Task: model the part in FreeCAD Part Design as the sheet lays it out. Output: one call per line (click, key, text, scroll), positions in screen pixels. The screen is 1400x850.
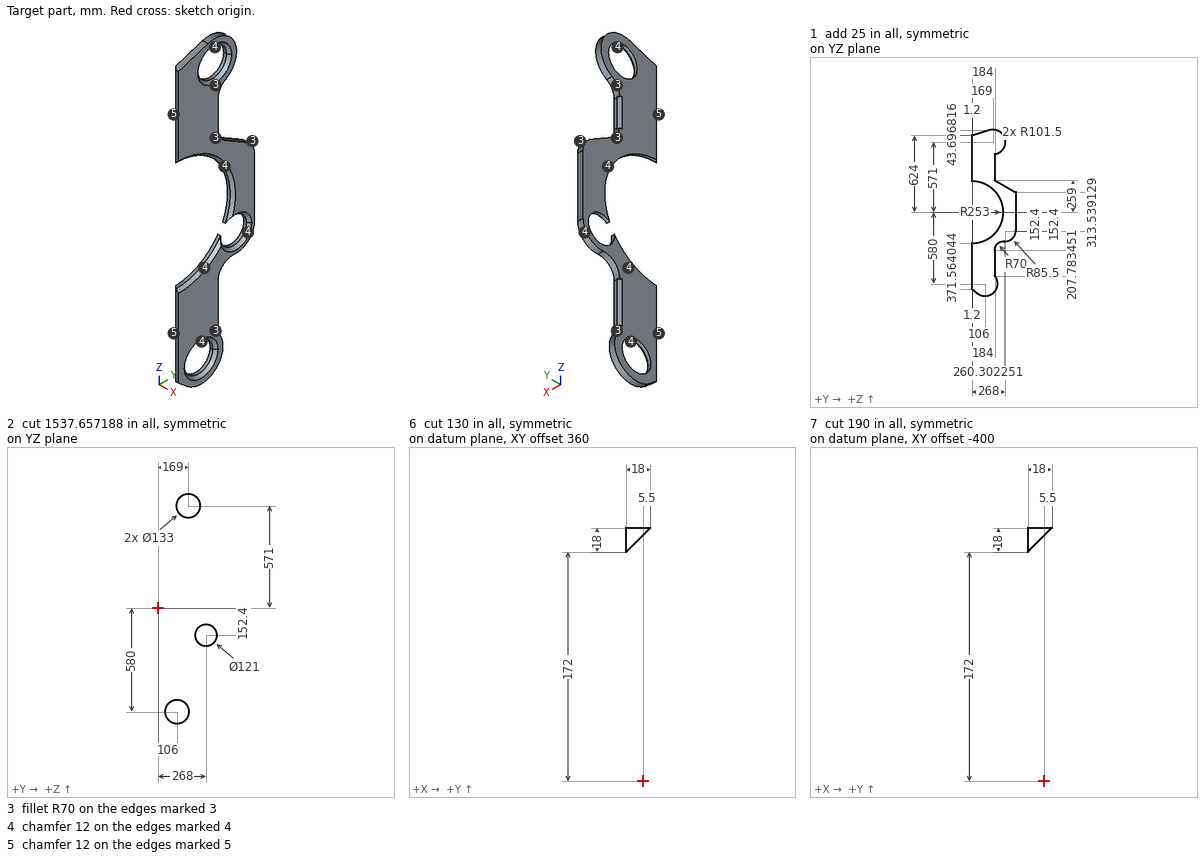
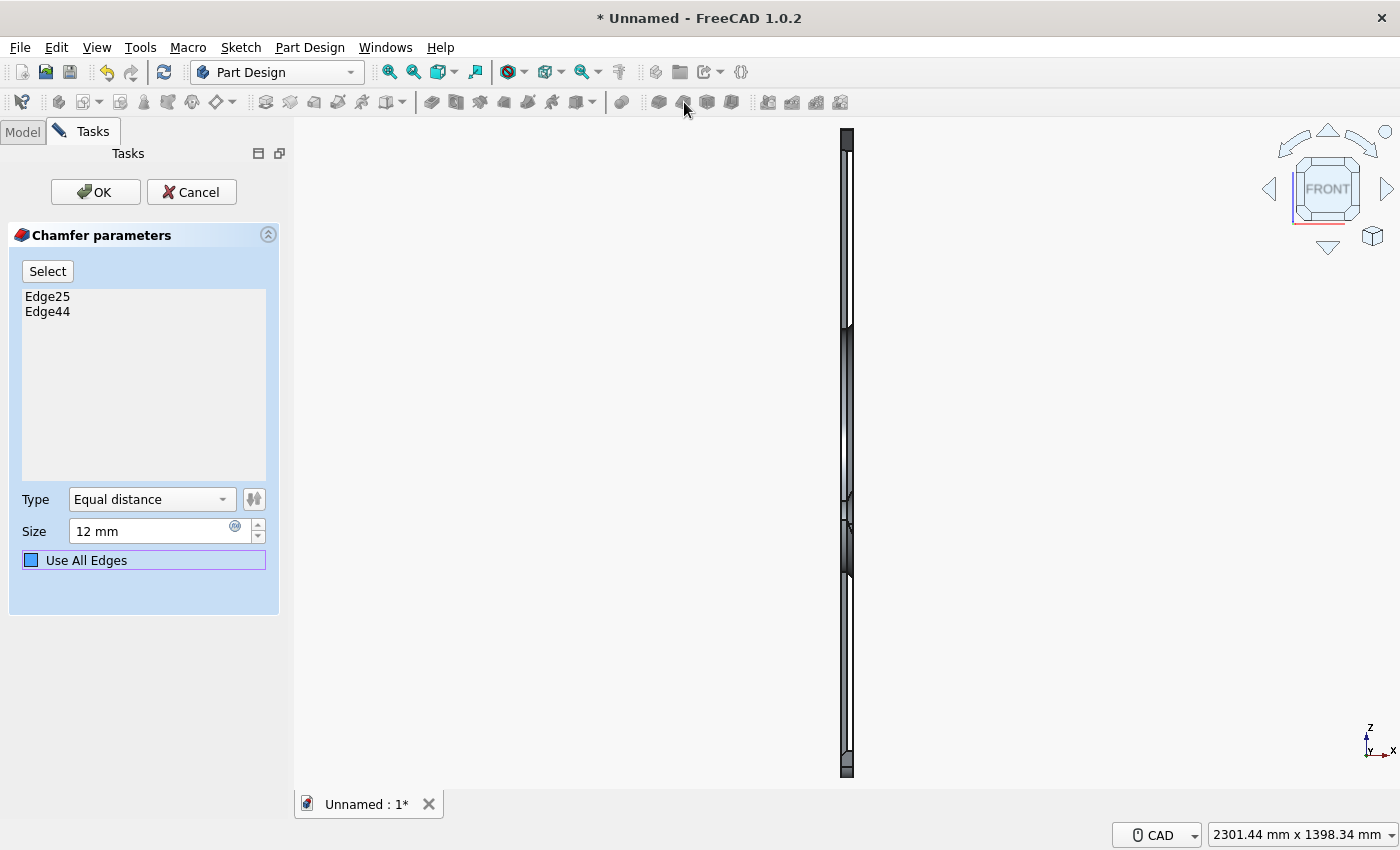
click(96, 192)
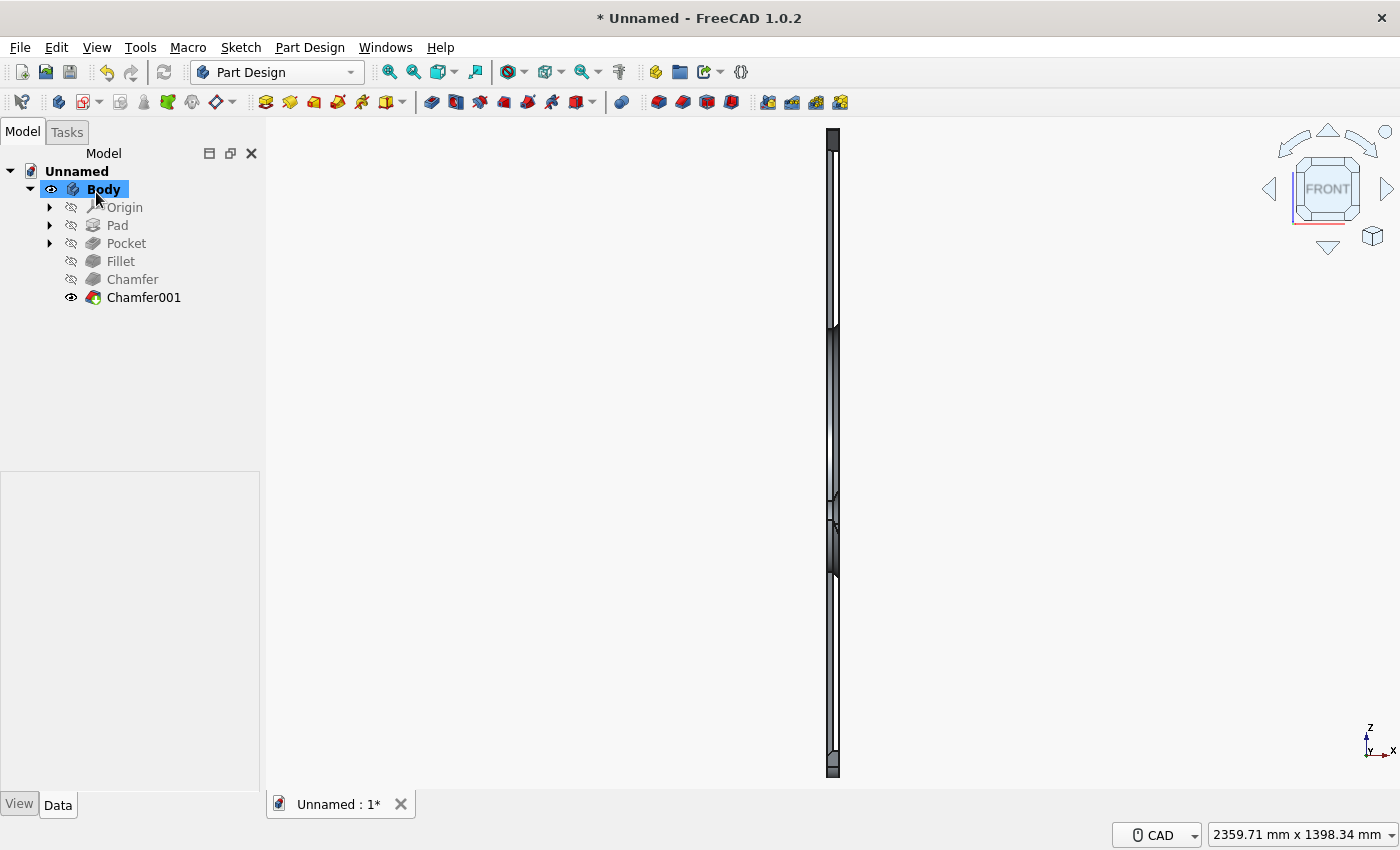
click(50, 207)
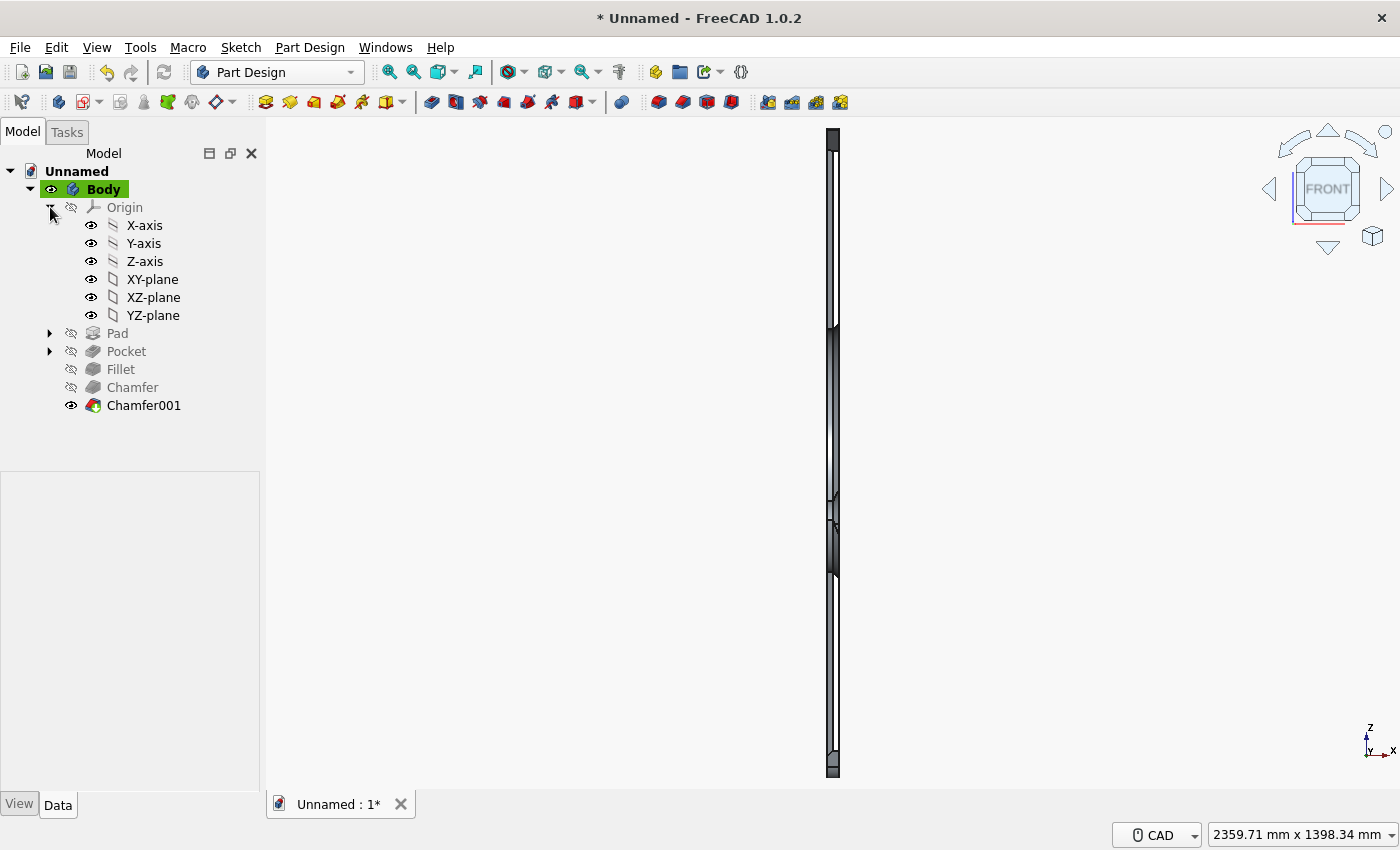
click(136, 279)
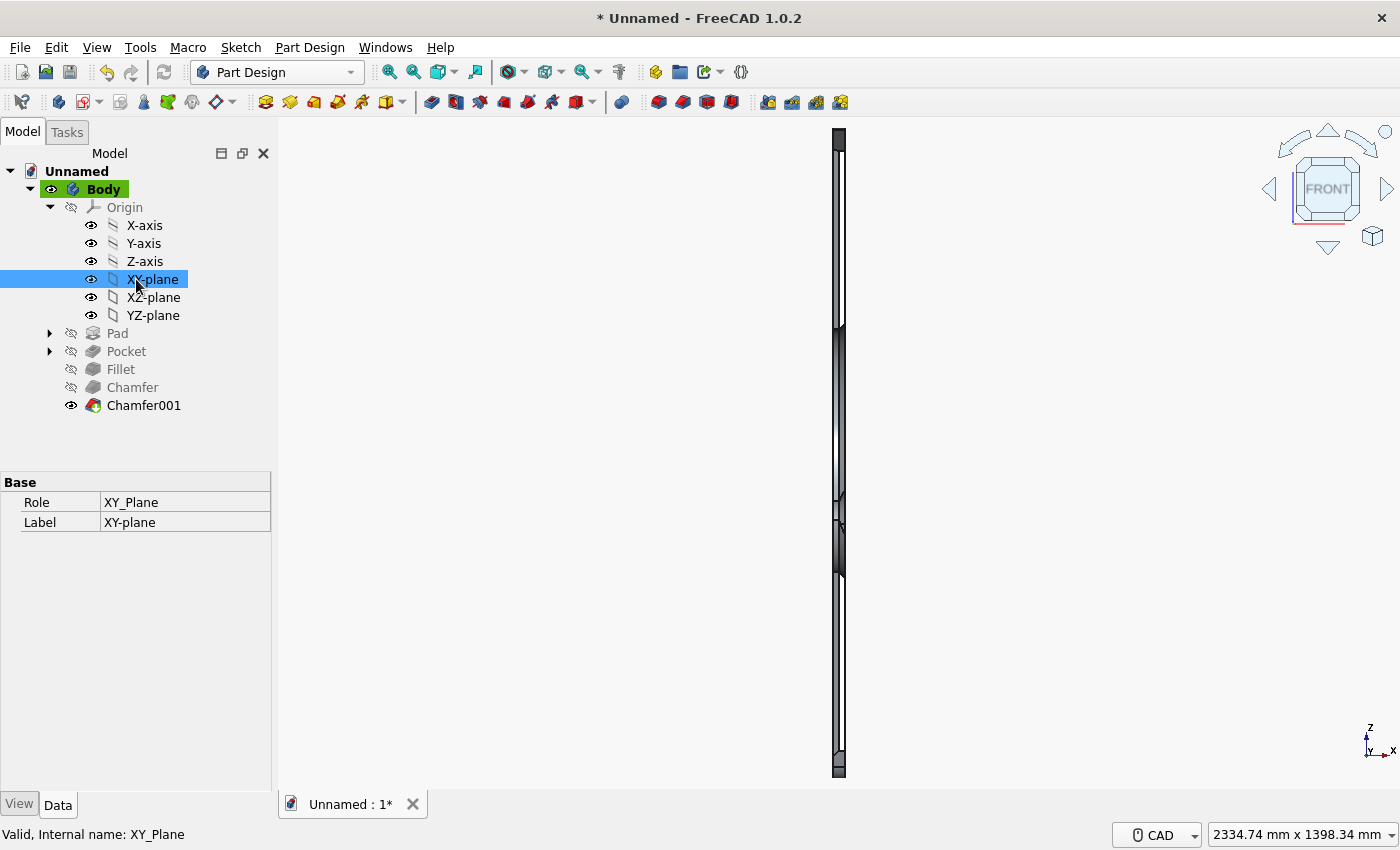
click(216, 102)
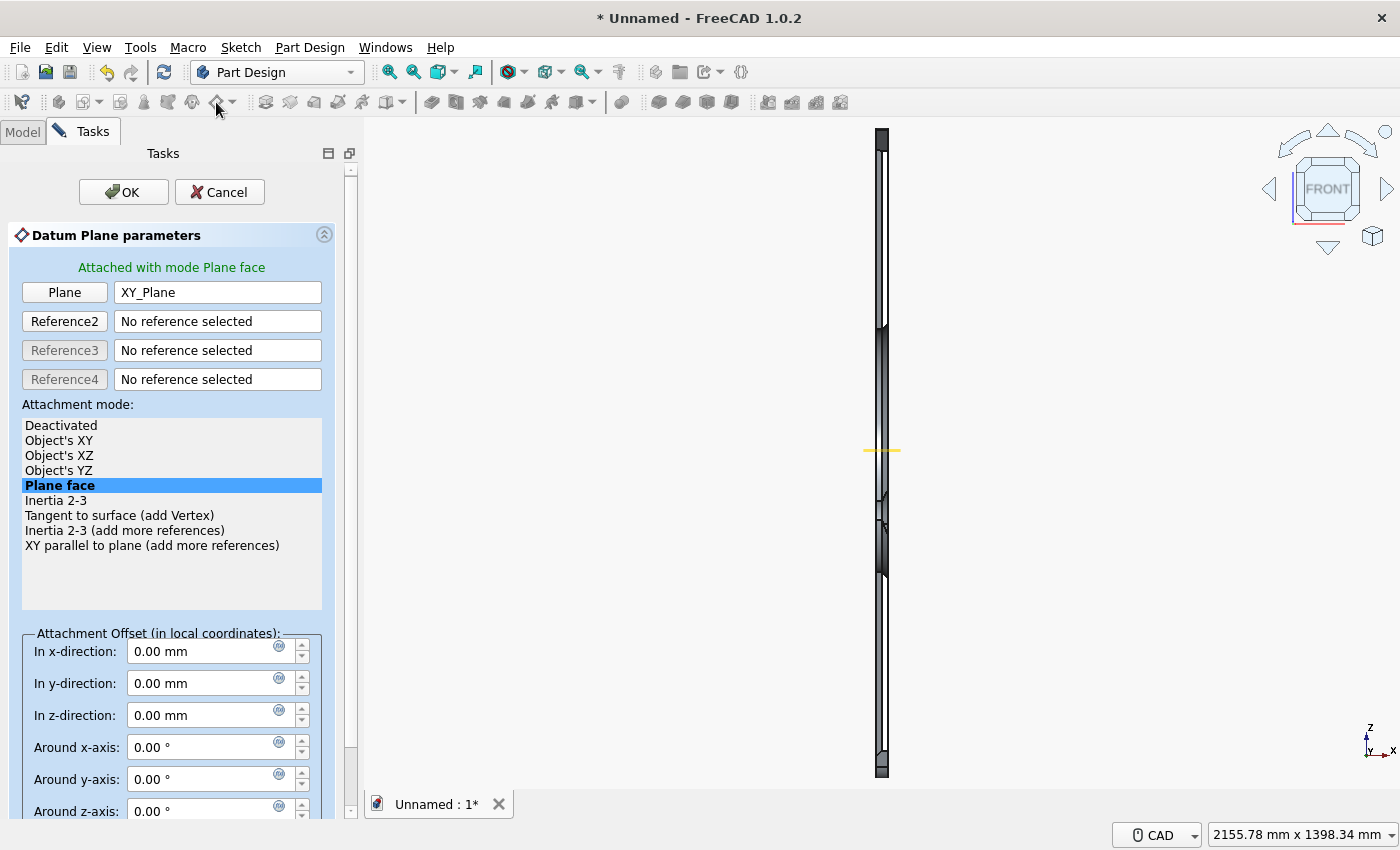
triple_click(210, 715)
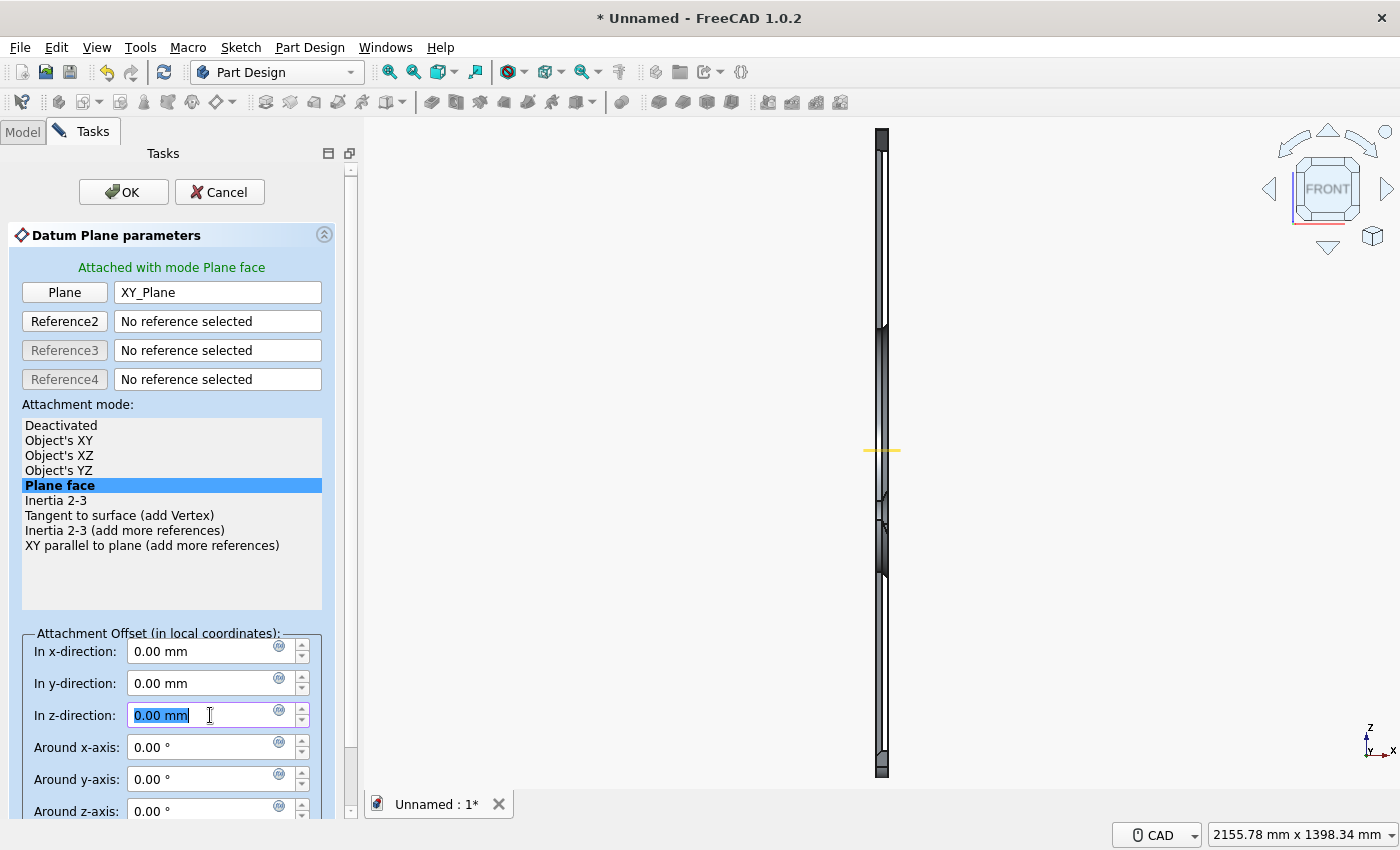
text(360)
key(Tab)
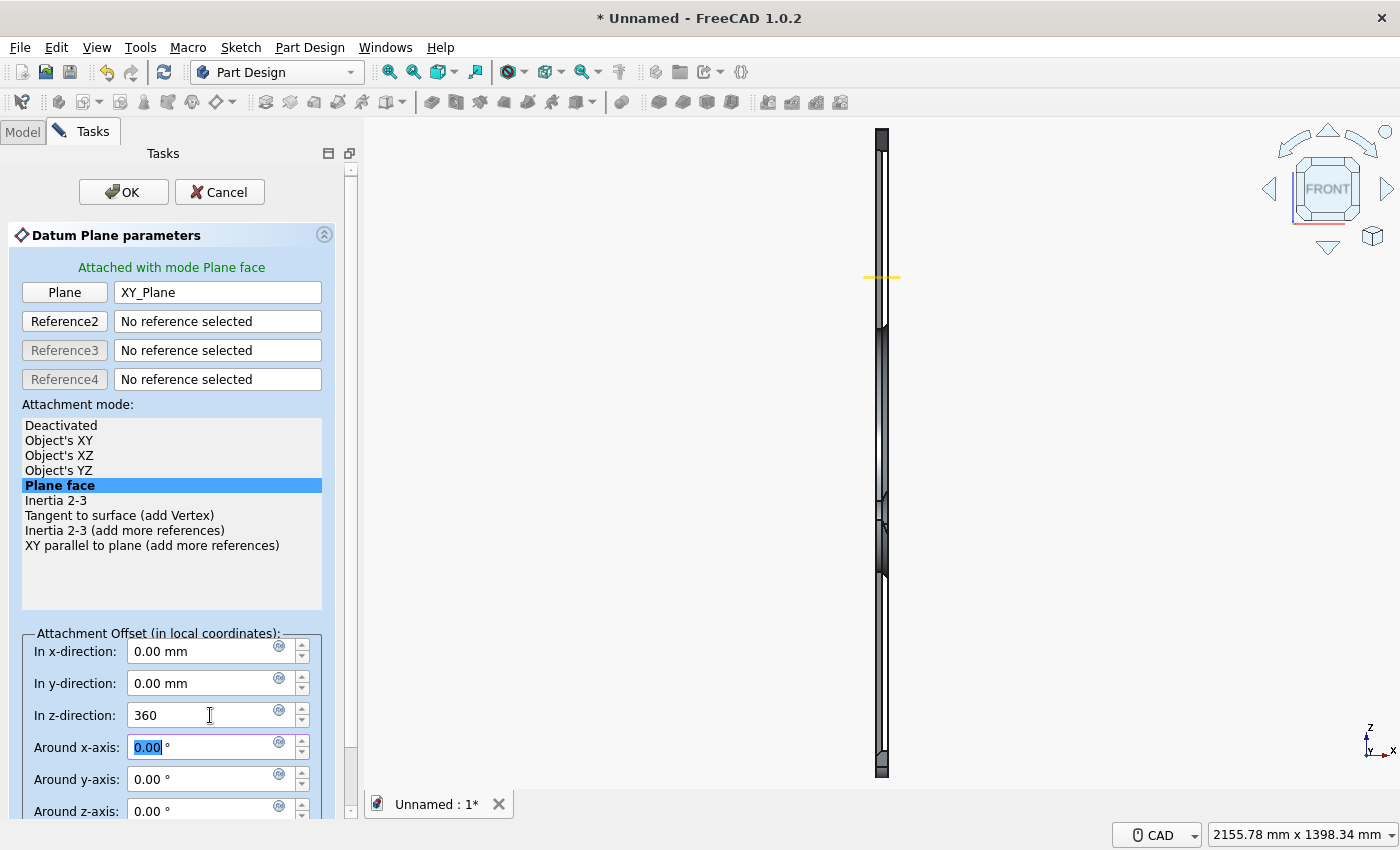
click(124, 192)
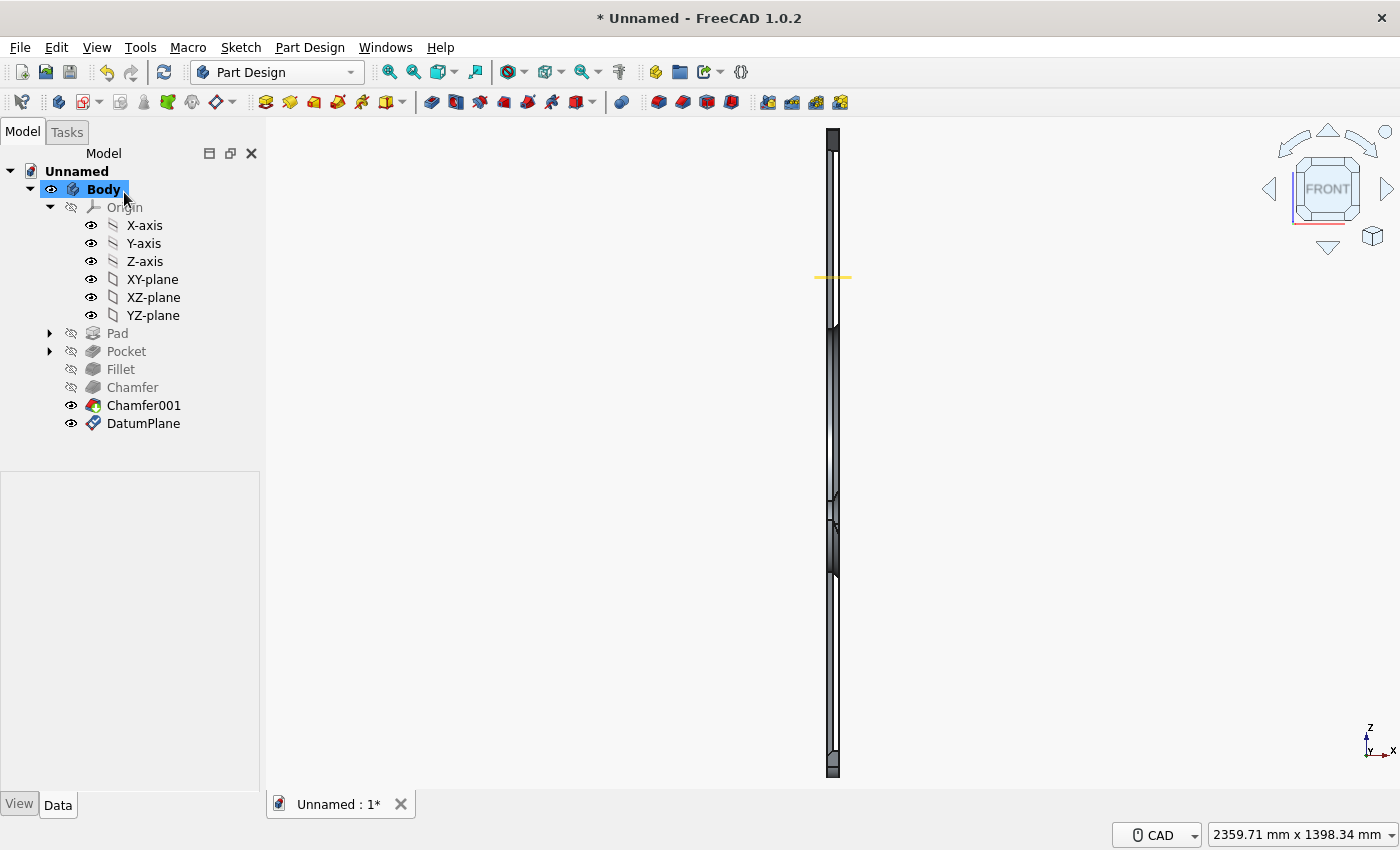
click(116, 423)